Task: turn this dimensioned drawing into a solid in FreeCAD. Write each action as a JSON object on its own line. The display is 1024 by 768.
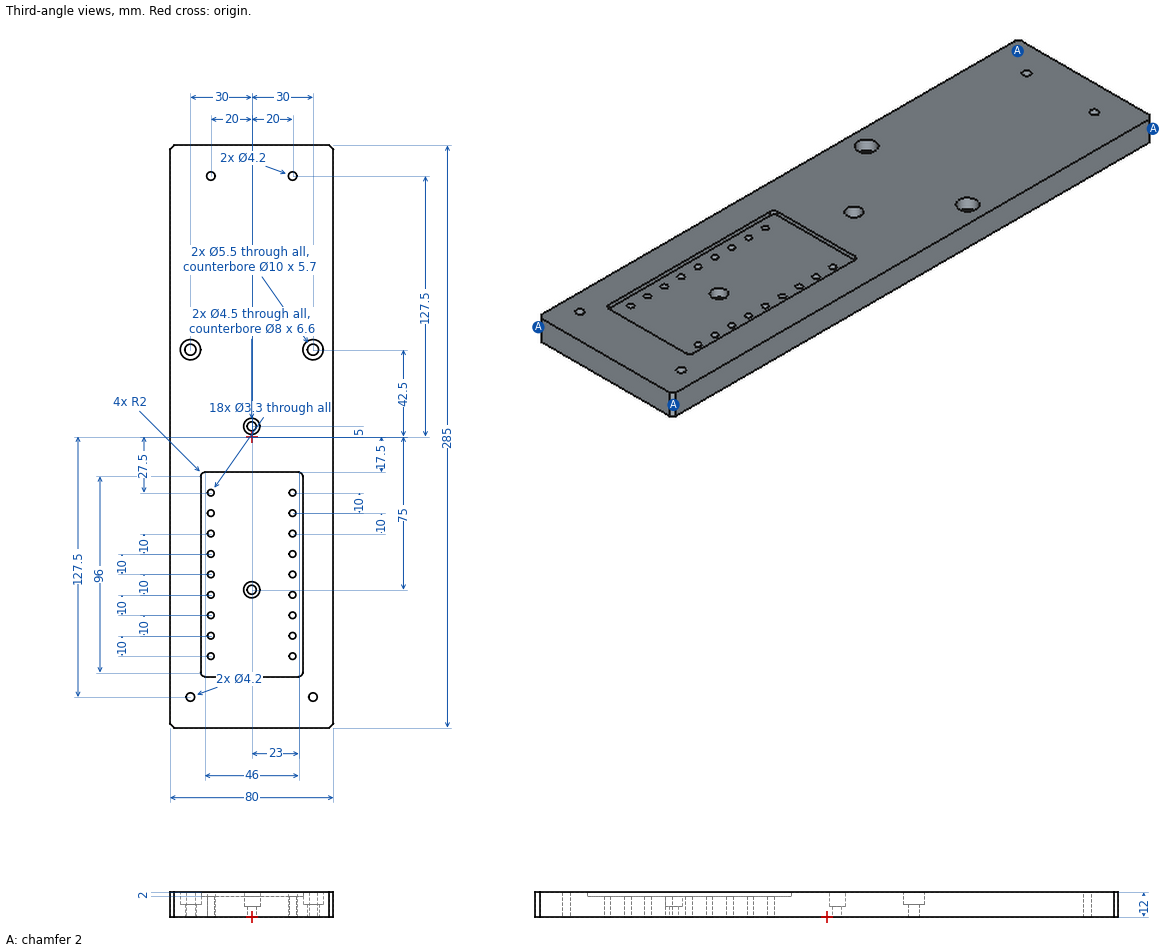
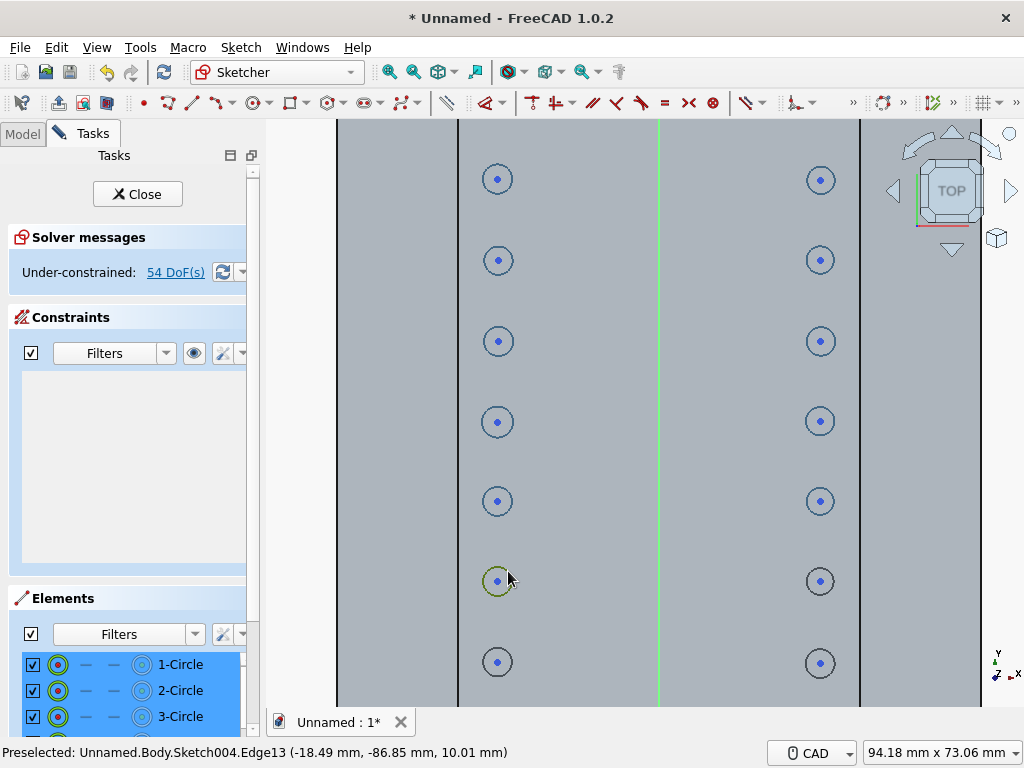
{"action": "left_click", "coordinate": [830, 572]}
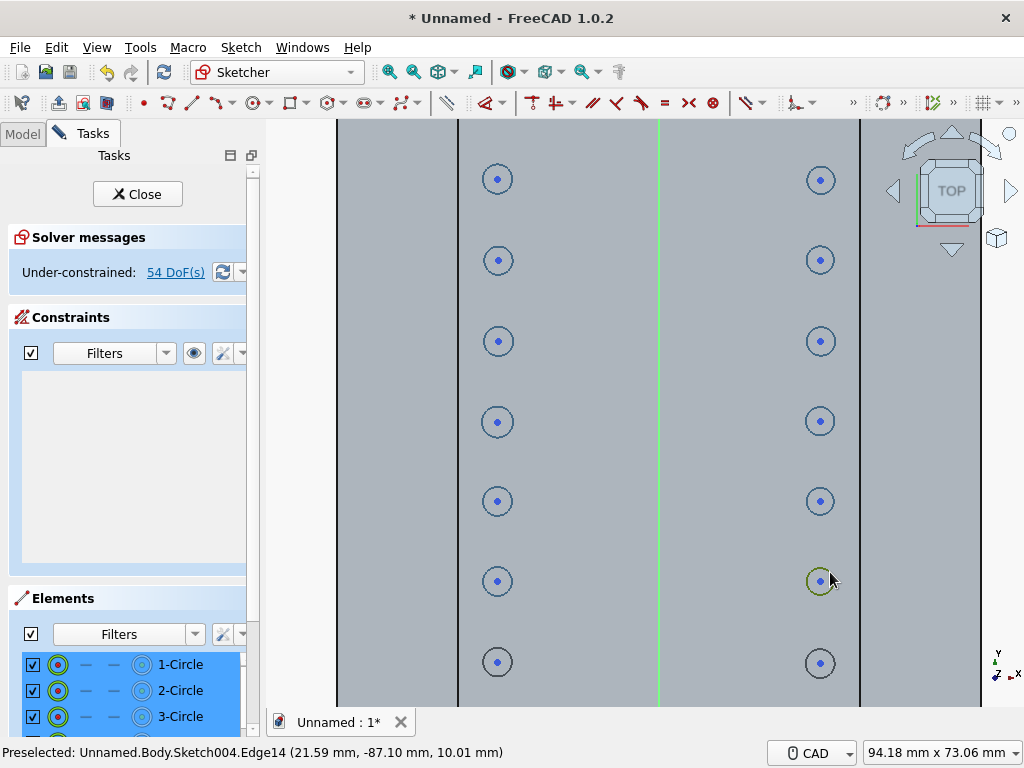
{"action": "left_click", "coordinate": [508, 652]}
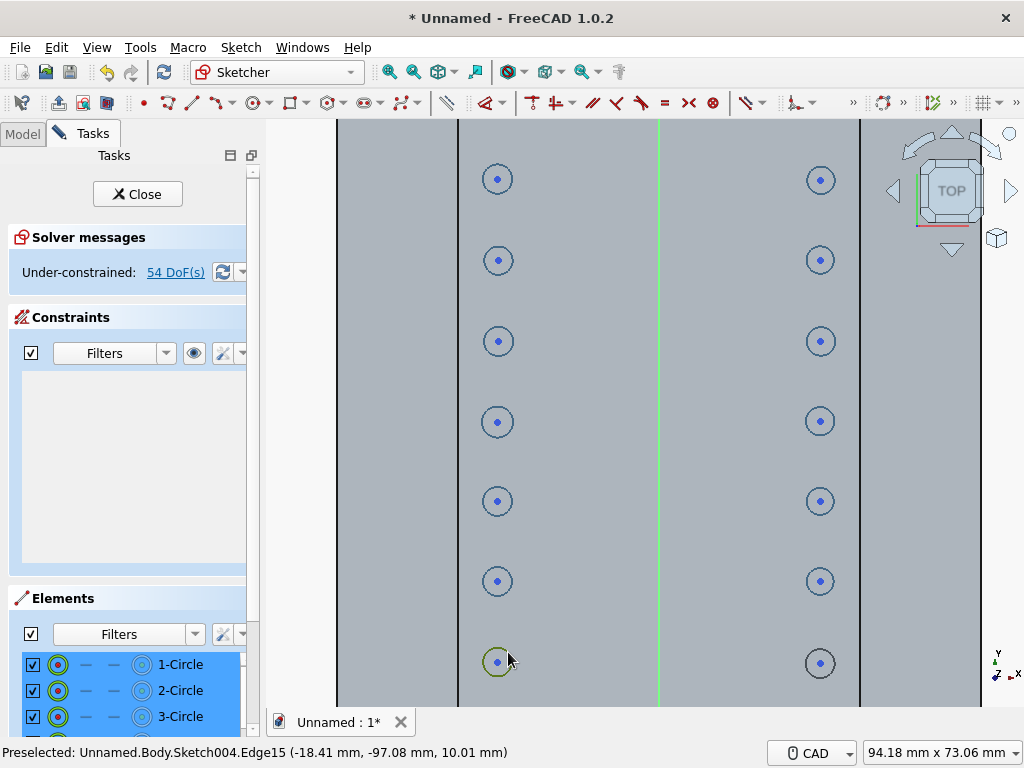
{"action": "left_click", "coordinate": [830, 653]}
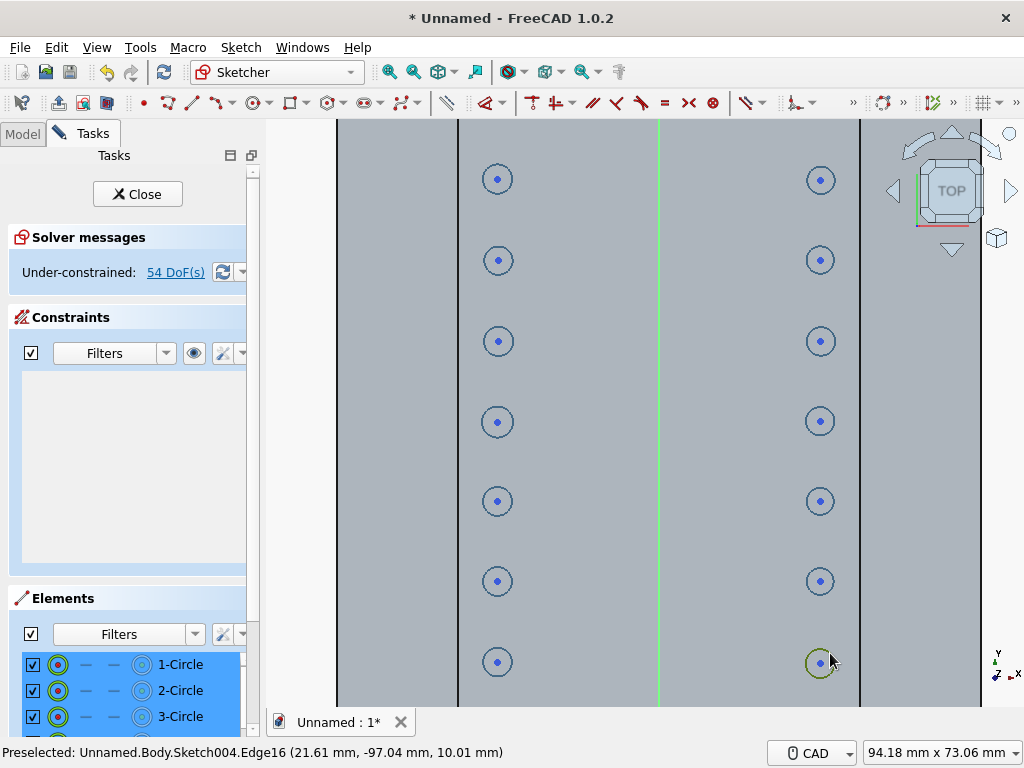
{"action": "scroll", "coordinate": [509, 493], "scroll_direction": "down", "scroll_amount": 4}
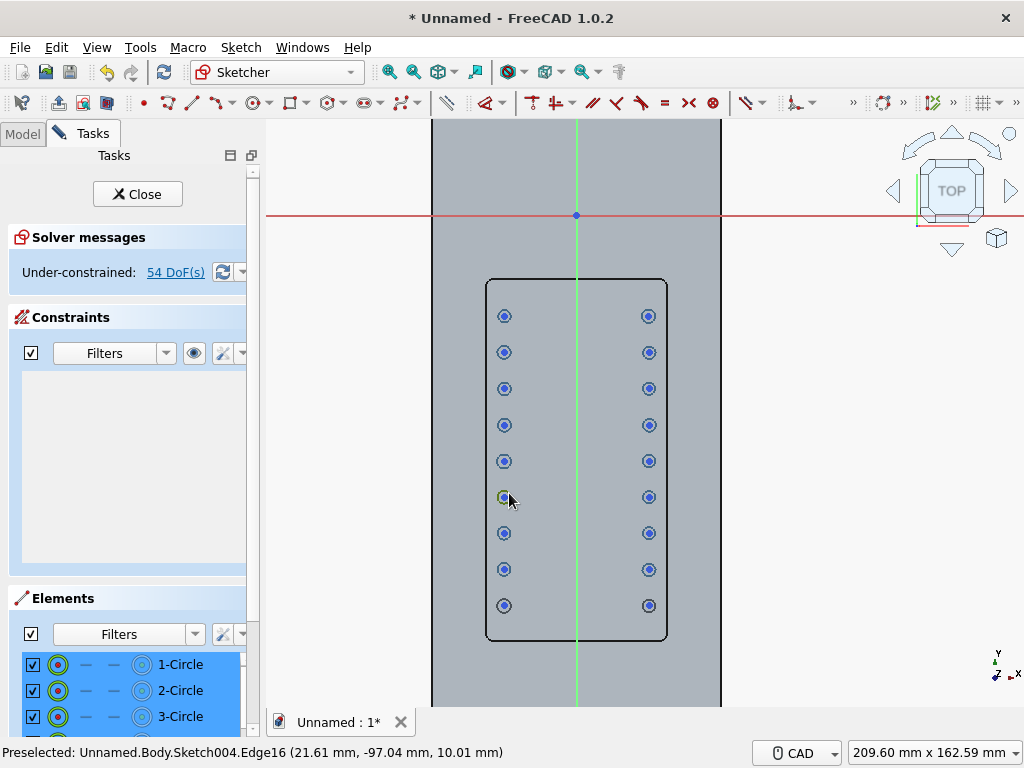
{"action": "scroll", "coordinate": [509, 601], "scroll_direction": "up", "scroll_amount": 4}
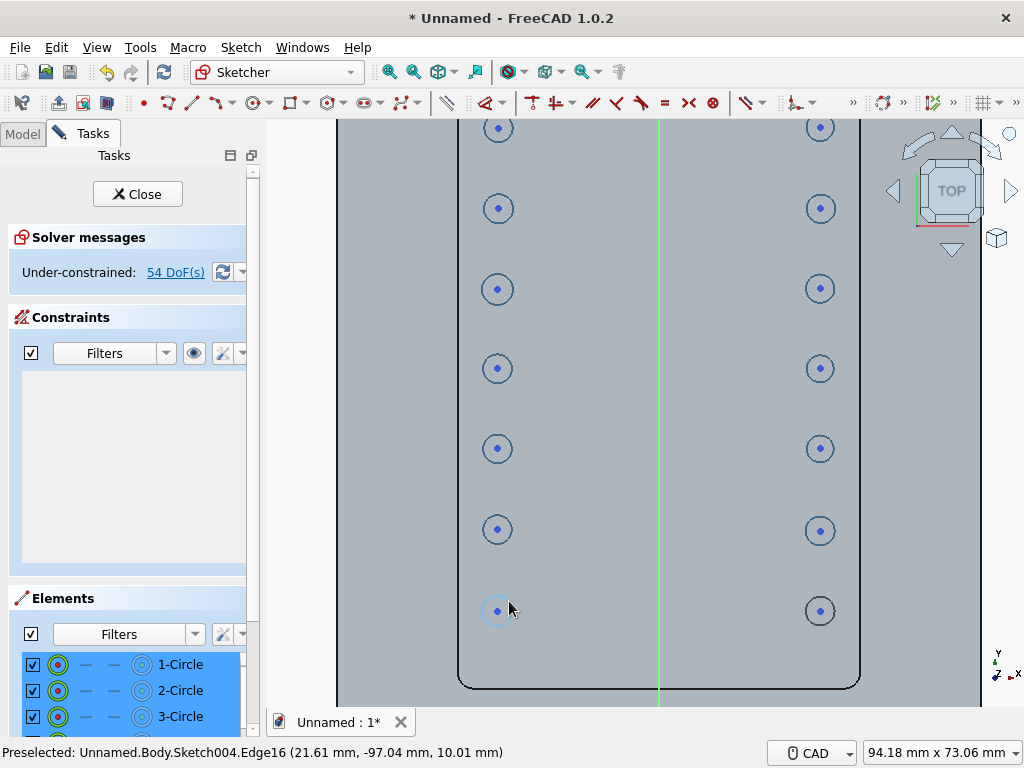
{"action": "left_click", "coordinate": [508, 600]}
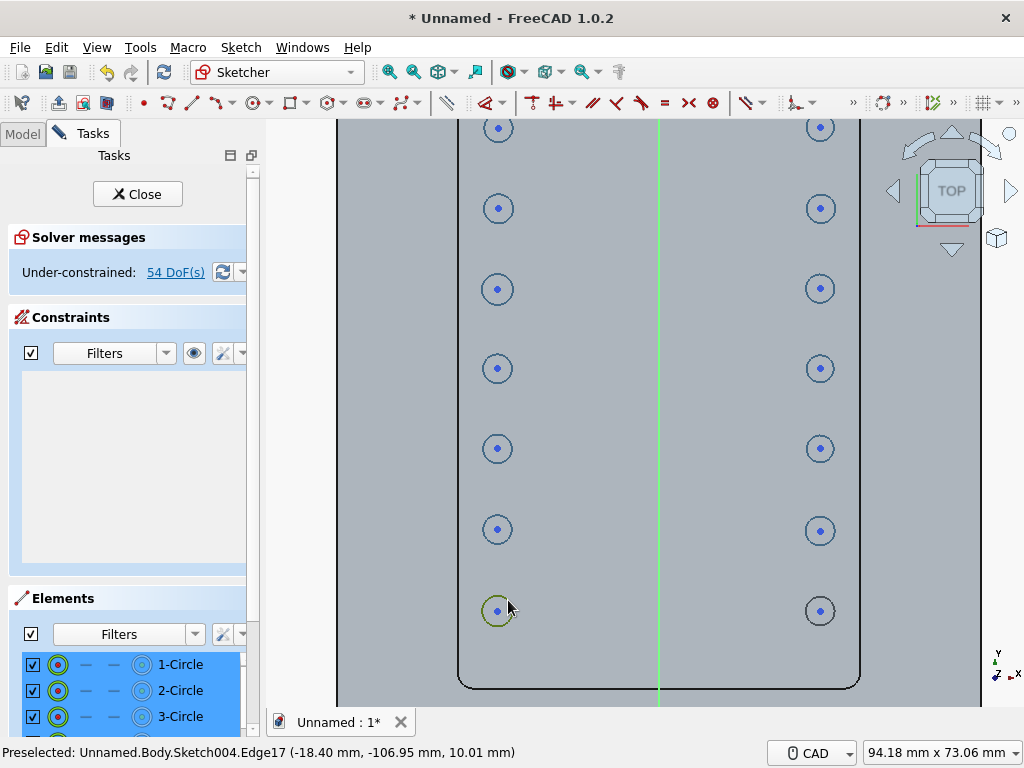
{"action": "left_click", "coordinate": [830, 601]}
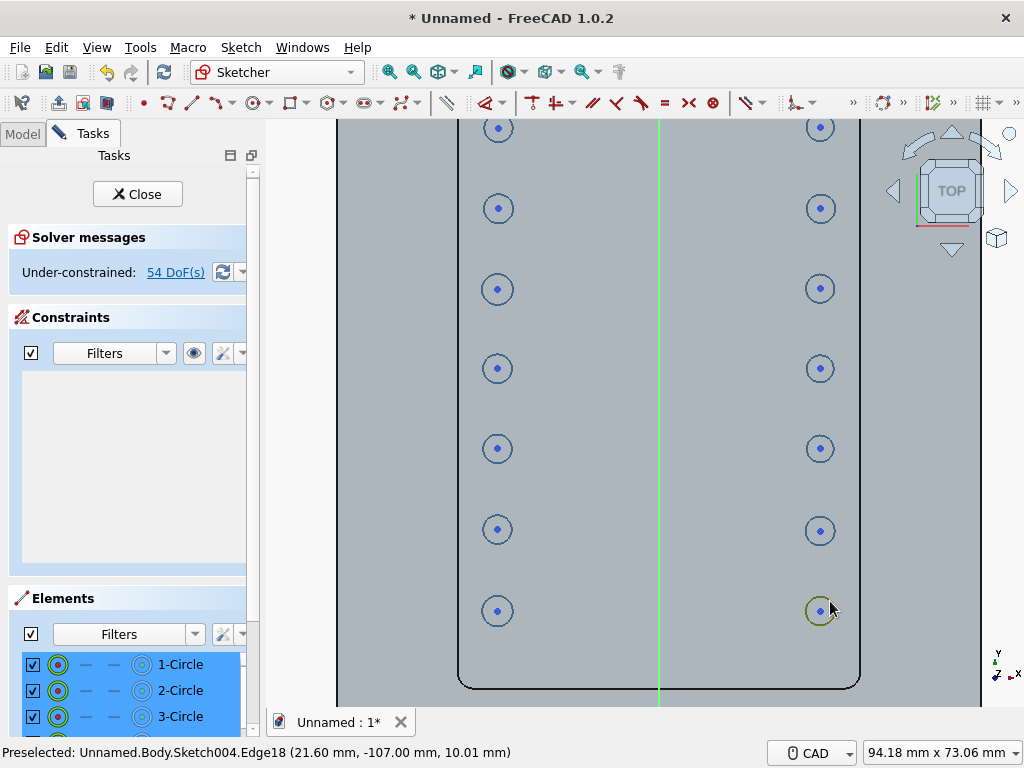
{"action": "left_click", "coordinate": [666, 104]}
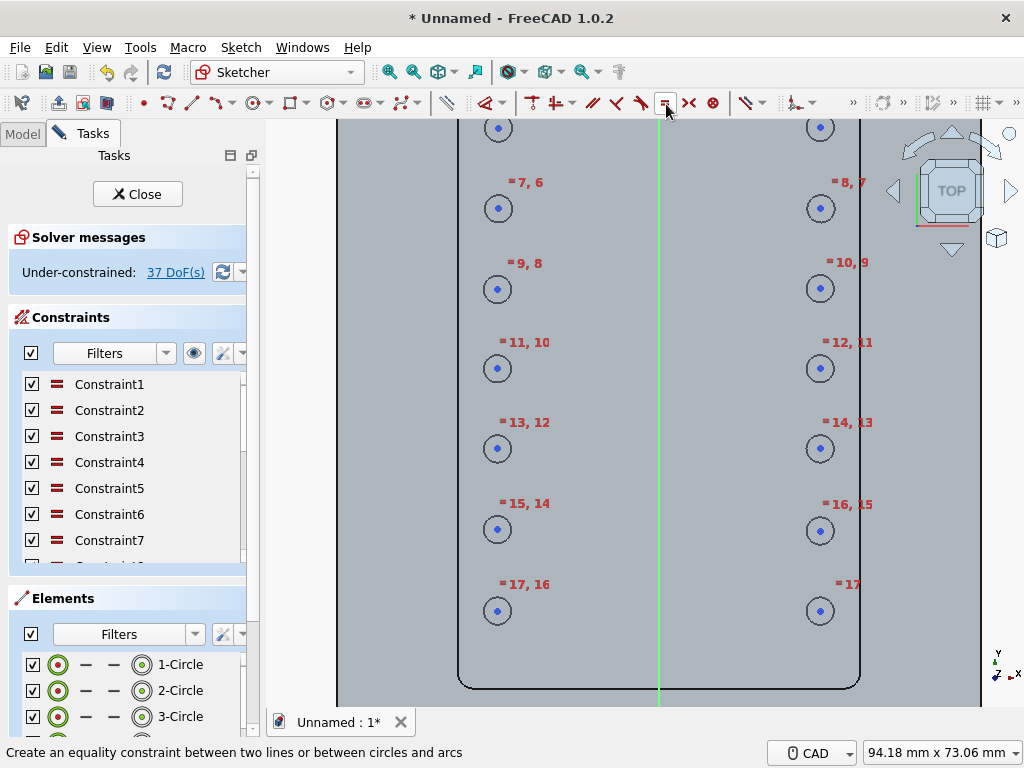
{"action": "scroll", "coordinate": [509, 601], "scroll_direction": "down", "scroll_amount": 4}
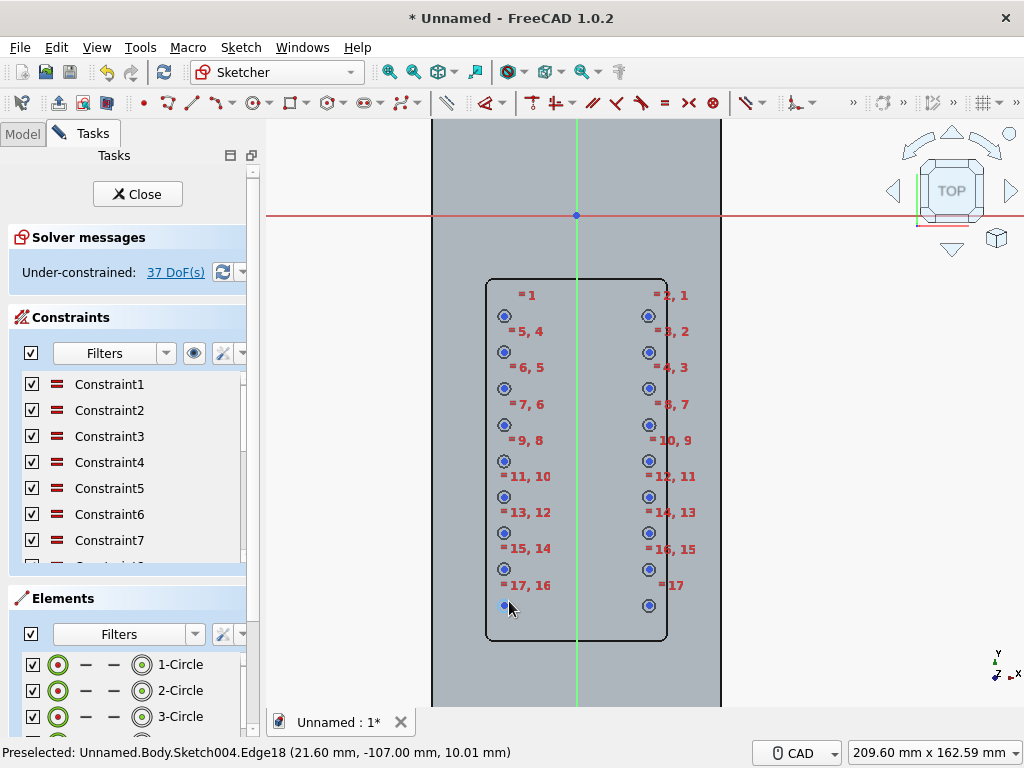
{"action": "left_click", "coordinate": [505, 316]}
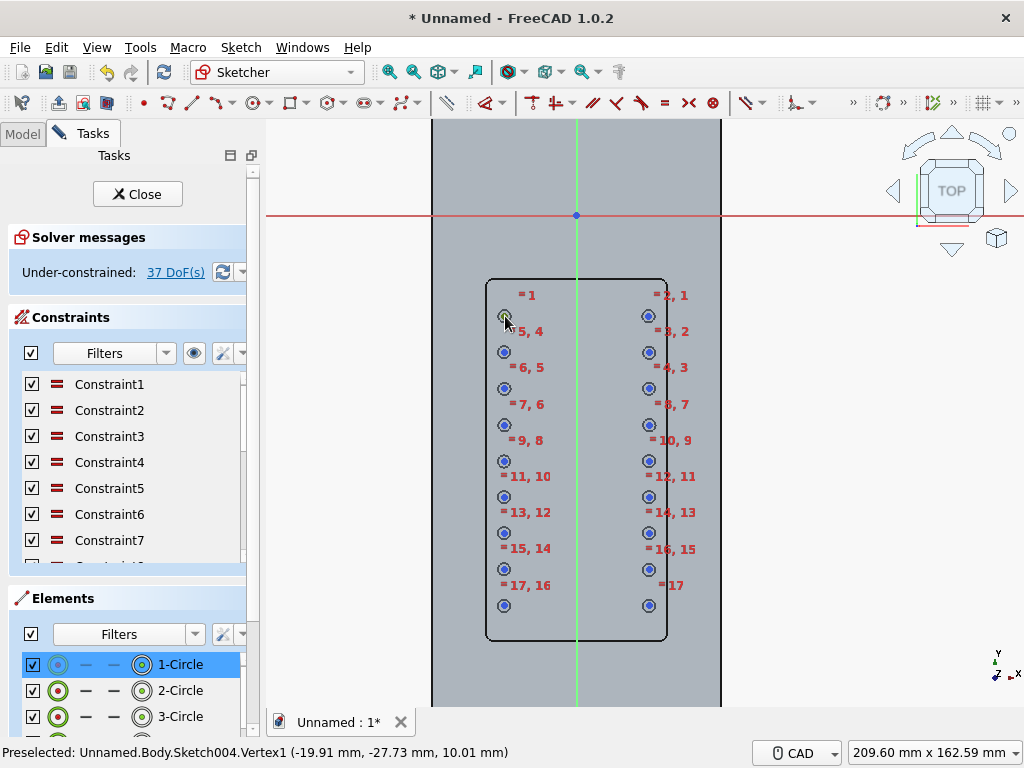
{"action": "left_click", "coordinate": [649, 316]}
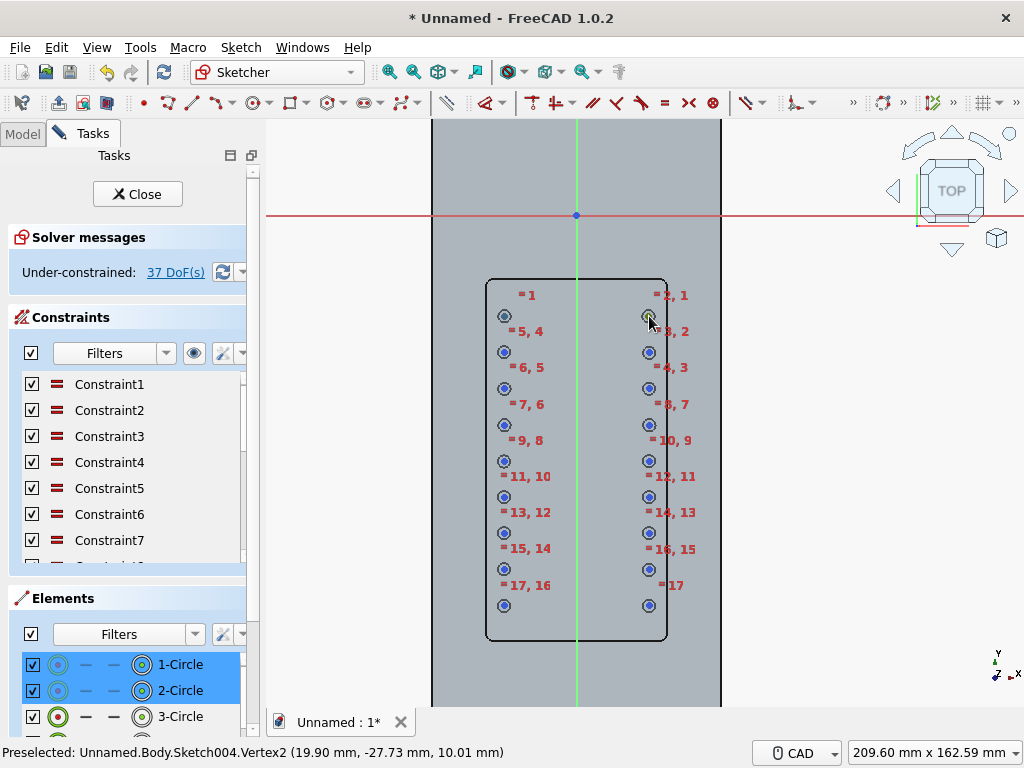
{"action": "key", "text": "h"}